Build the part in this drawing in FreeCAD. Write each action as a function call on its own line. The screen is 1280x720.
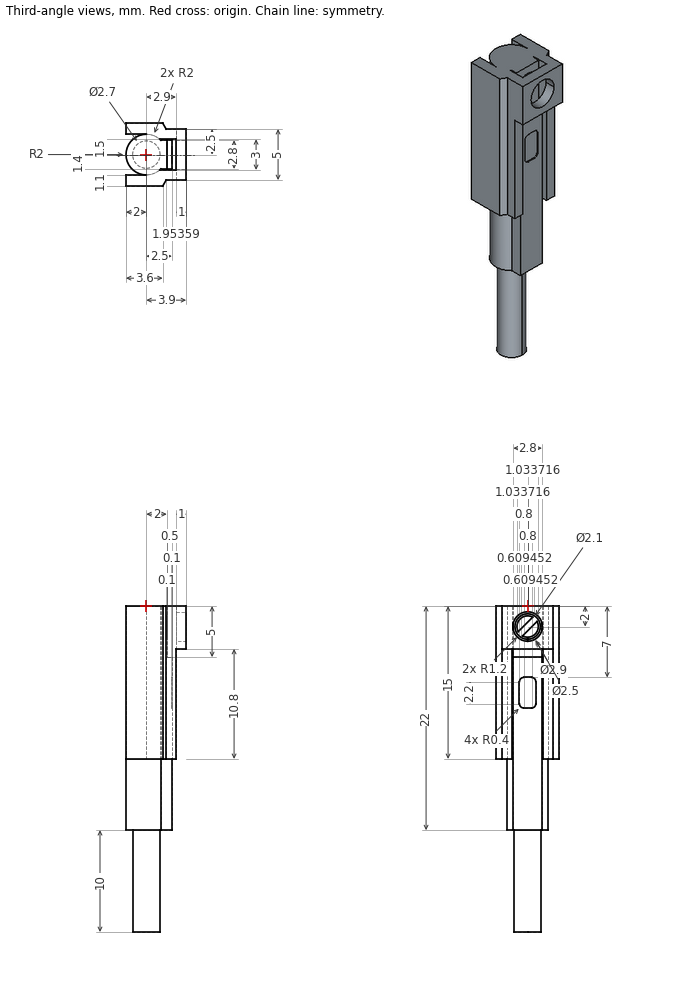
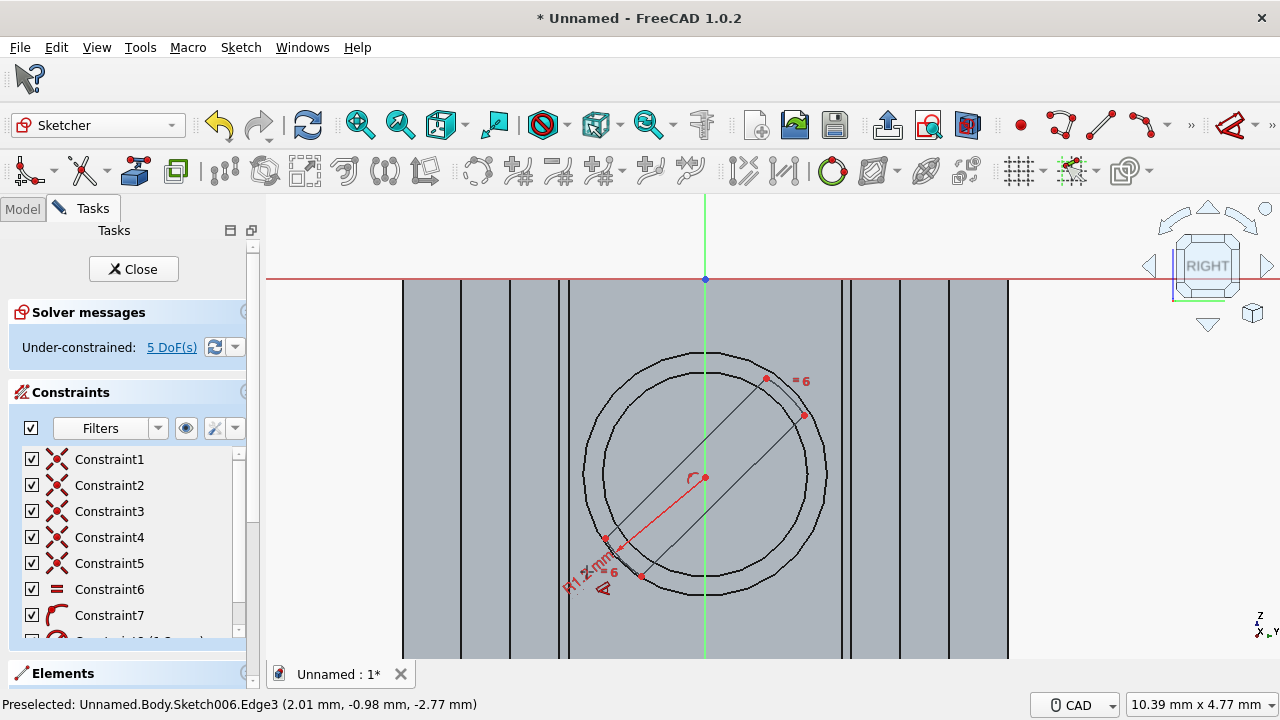
click(705, 478)
click(739, 378)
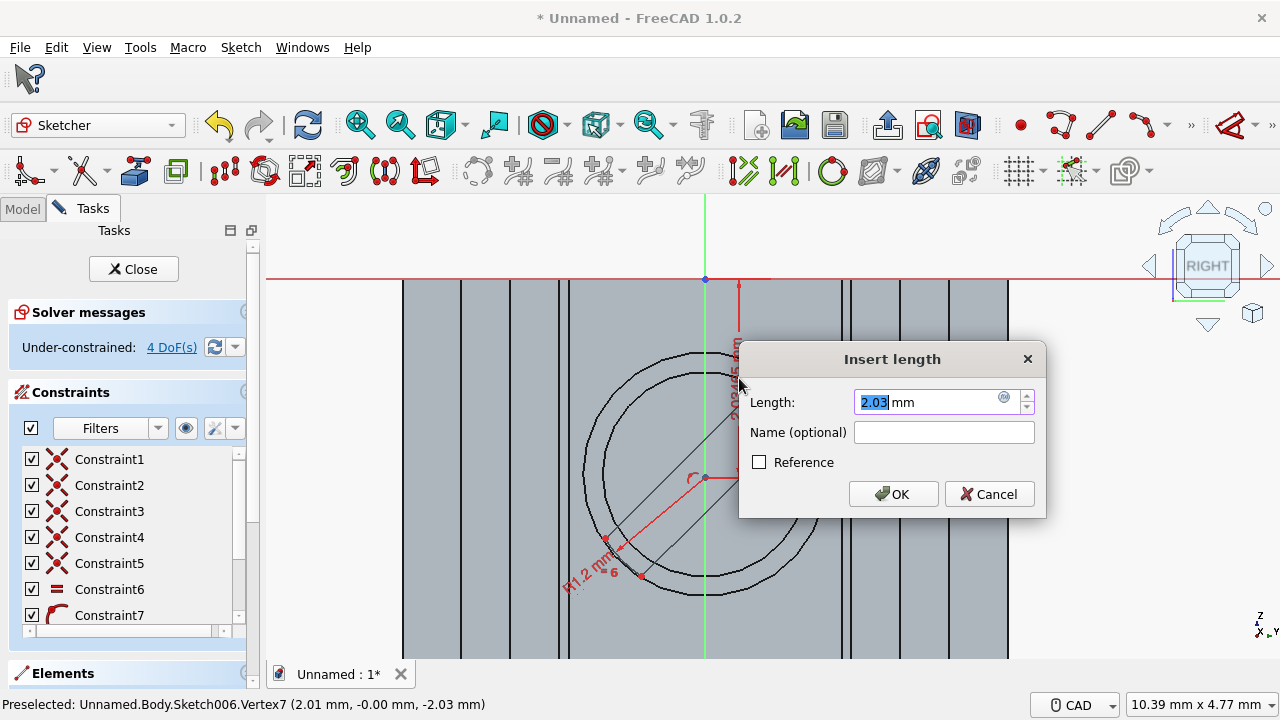
text(2)
key(Return)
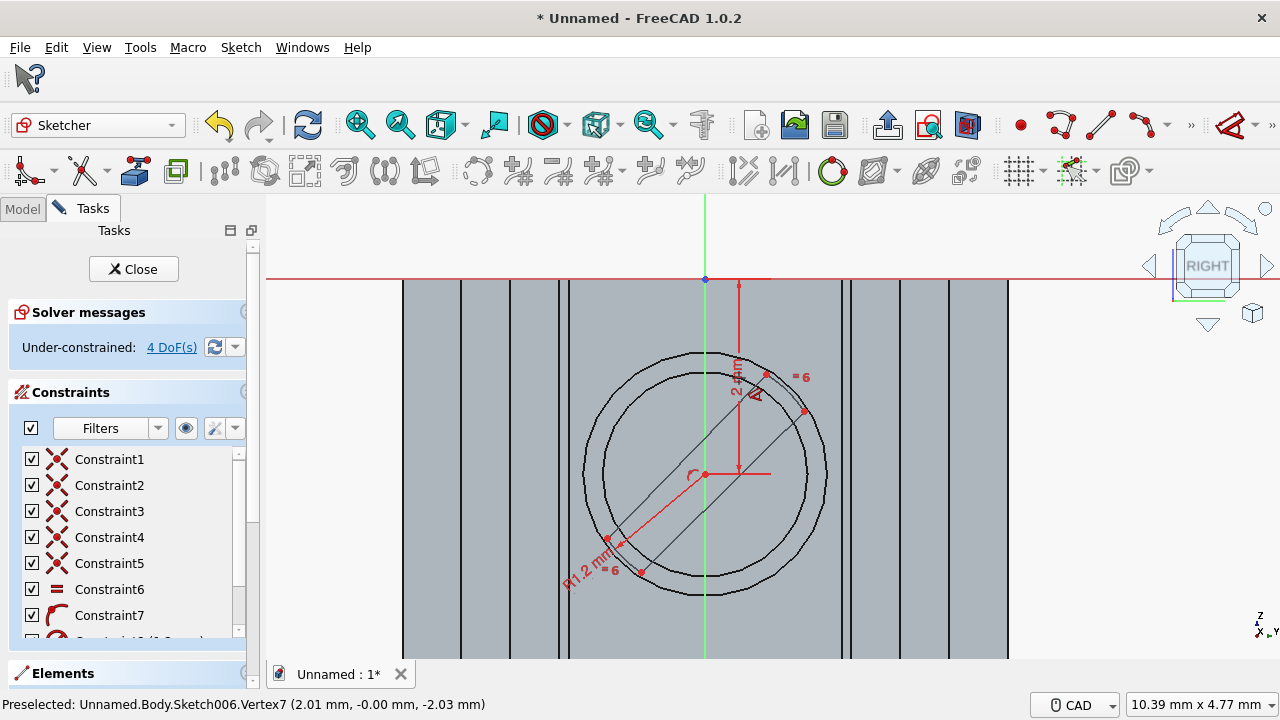
click(767, 375)
click(736, 245)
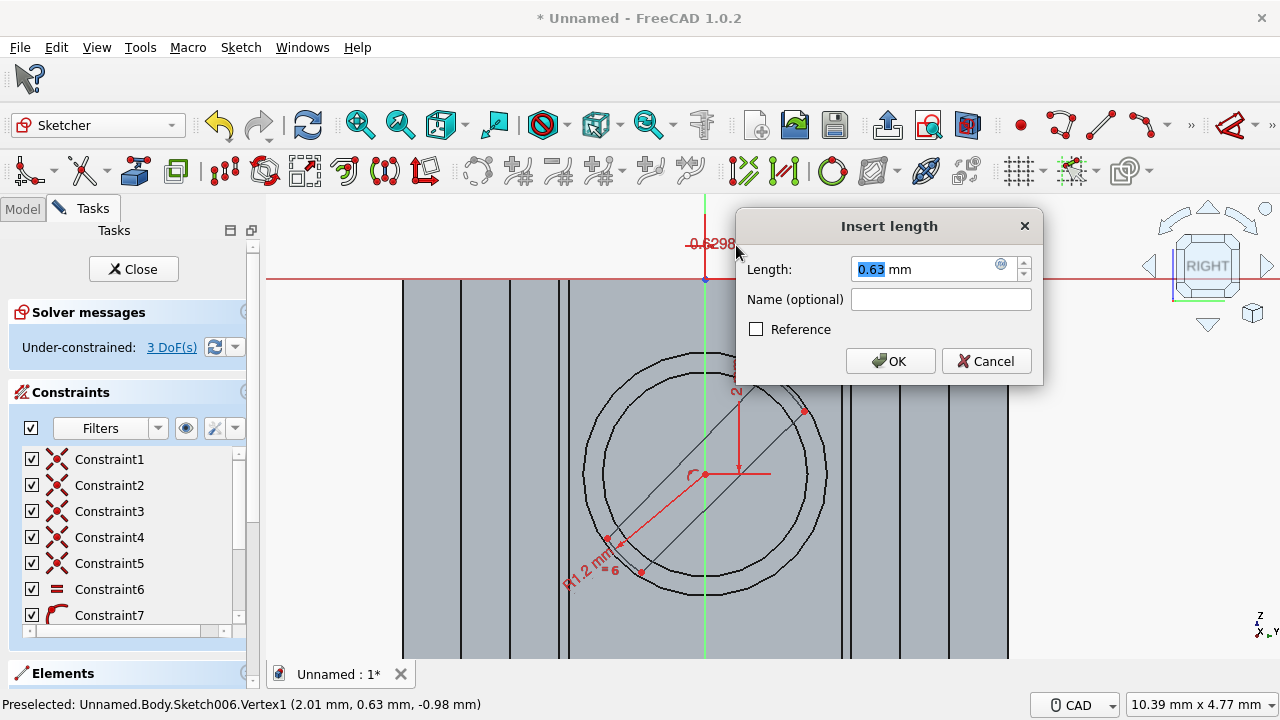
text(0.609452)
key(Return)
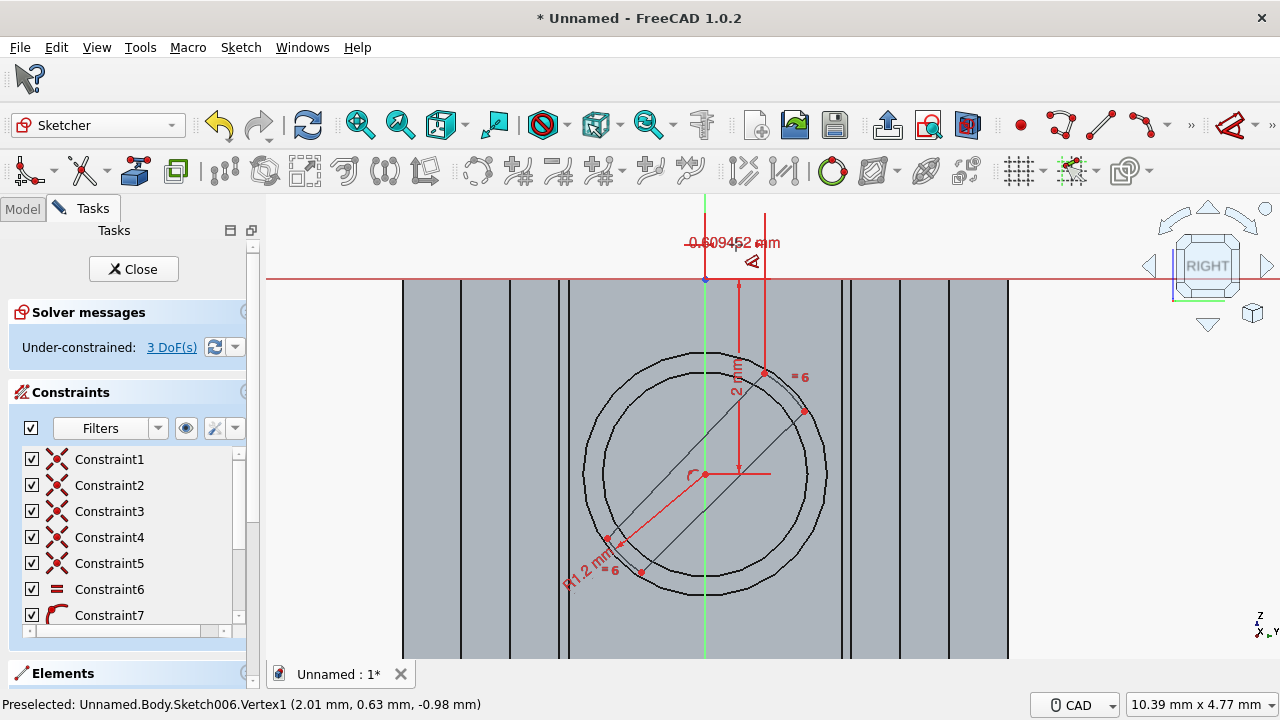
click(607, 539)
click(656, 245)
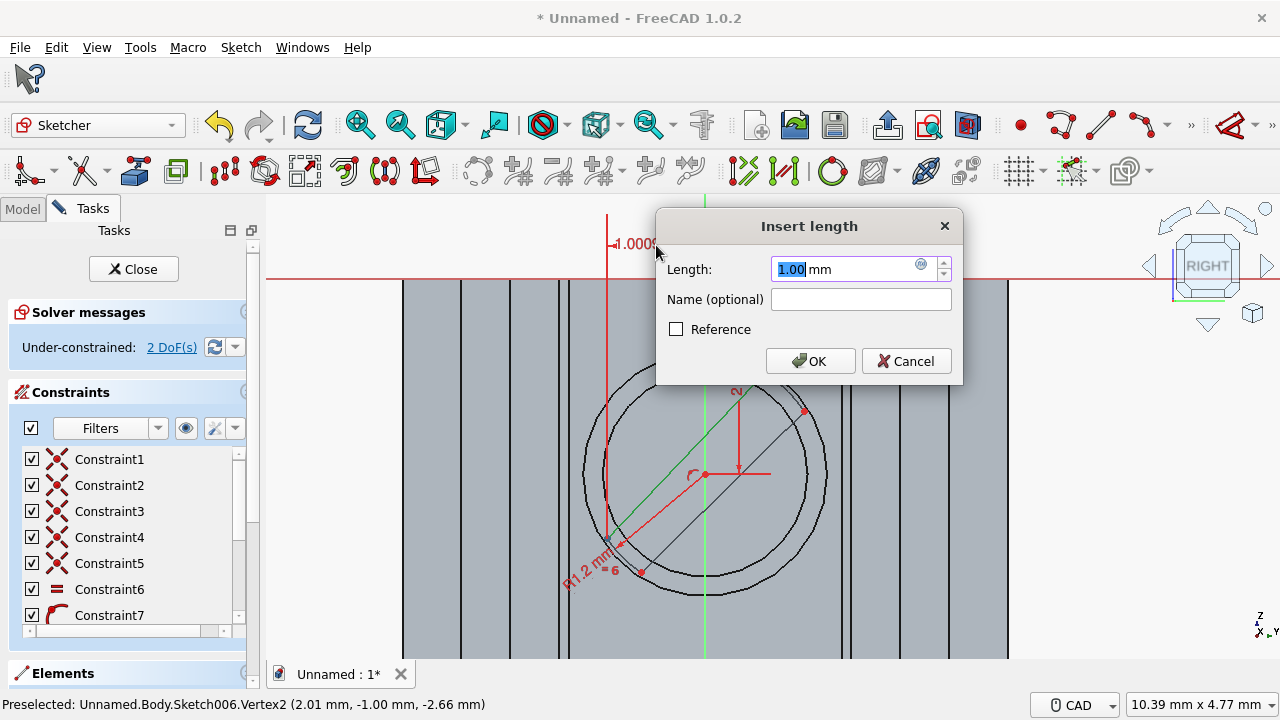
text(1.033716)
key(Return)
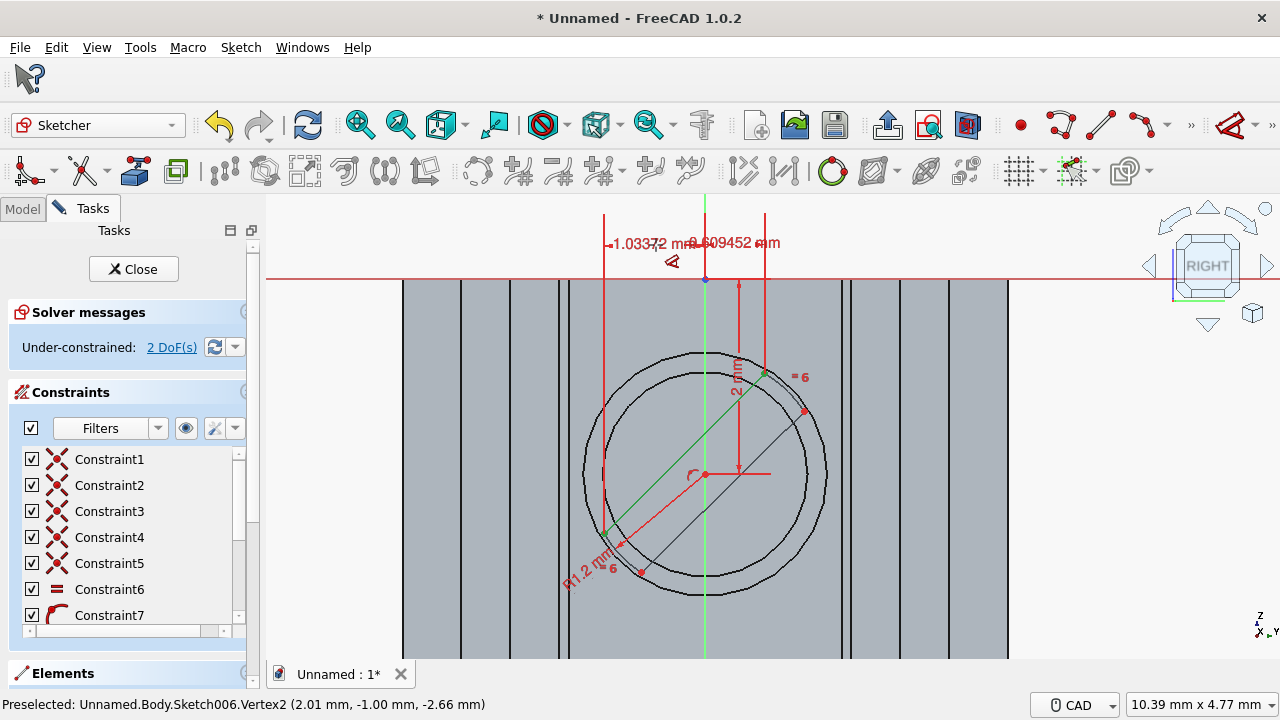
click(642, 573)
click(673, 607)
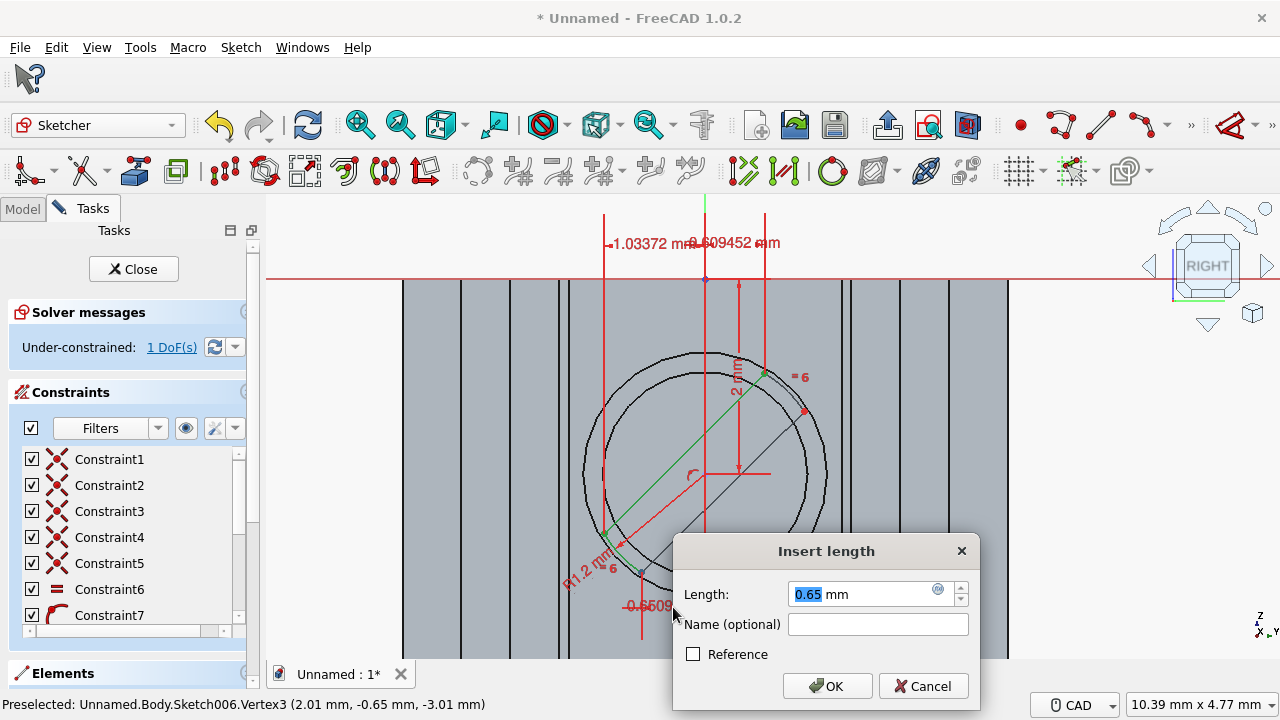
text(0.609452)
key(Return)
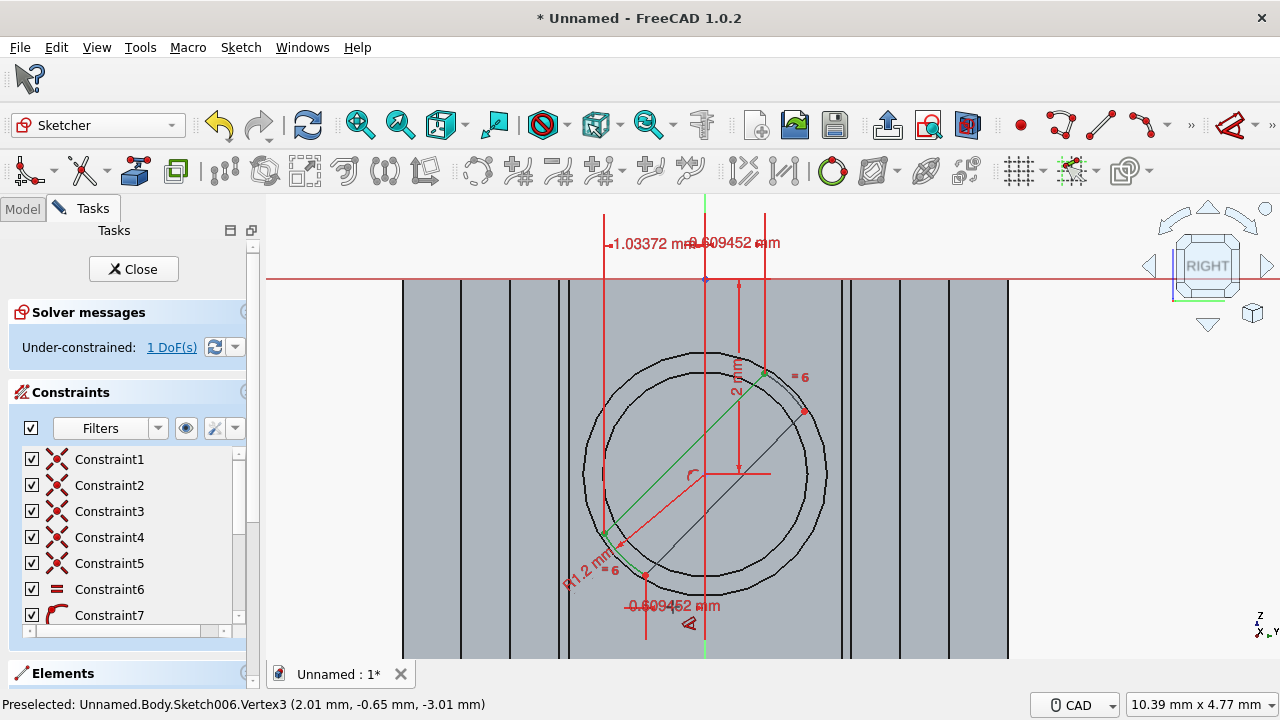
click(804, 412)
click(732, 446)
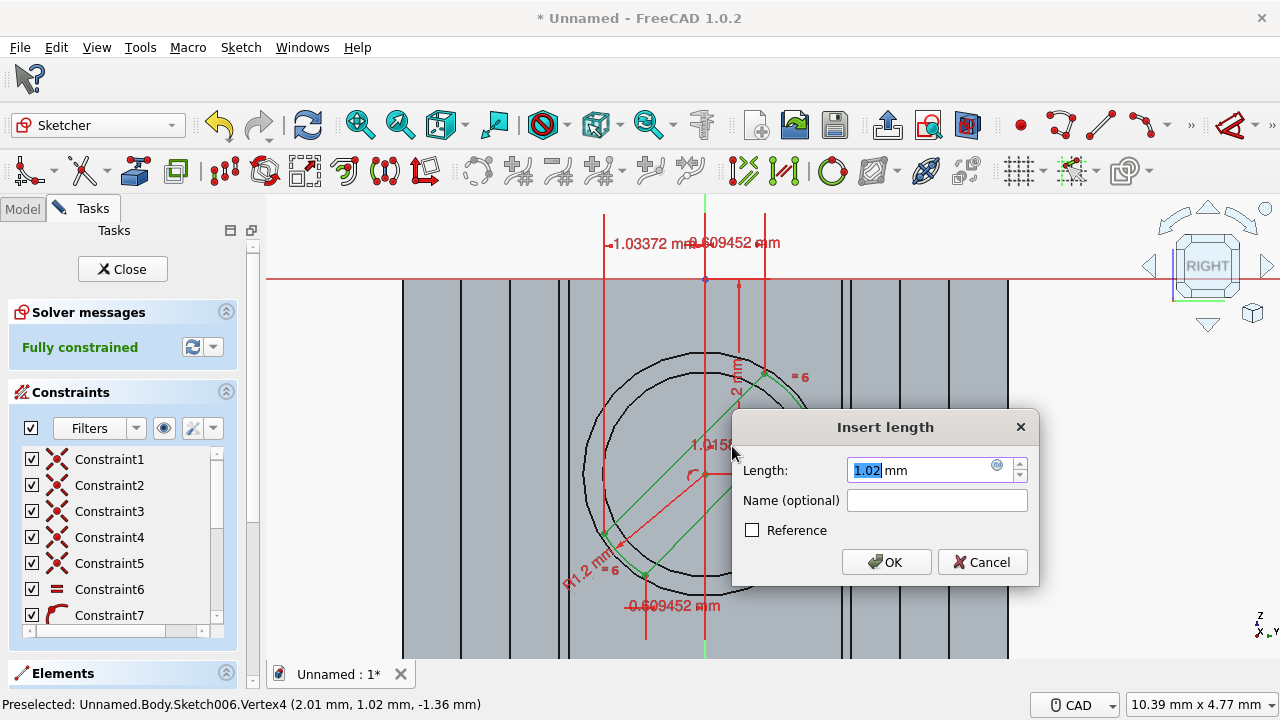
text(1.033716)
key(Return)
key(Escape)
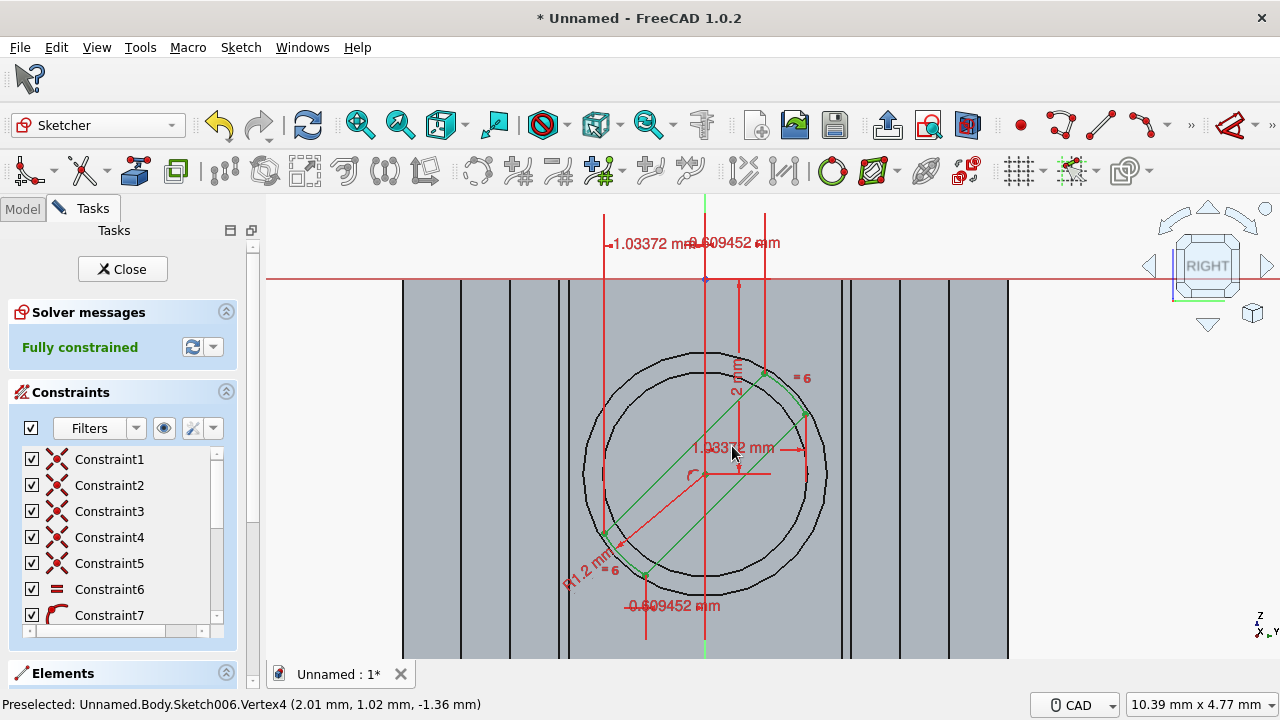
click(123, 269)